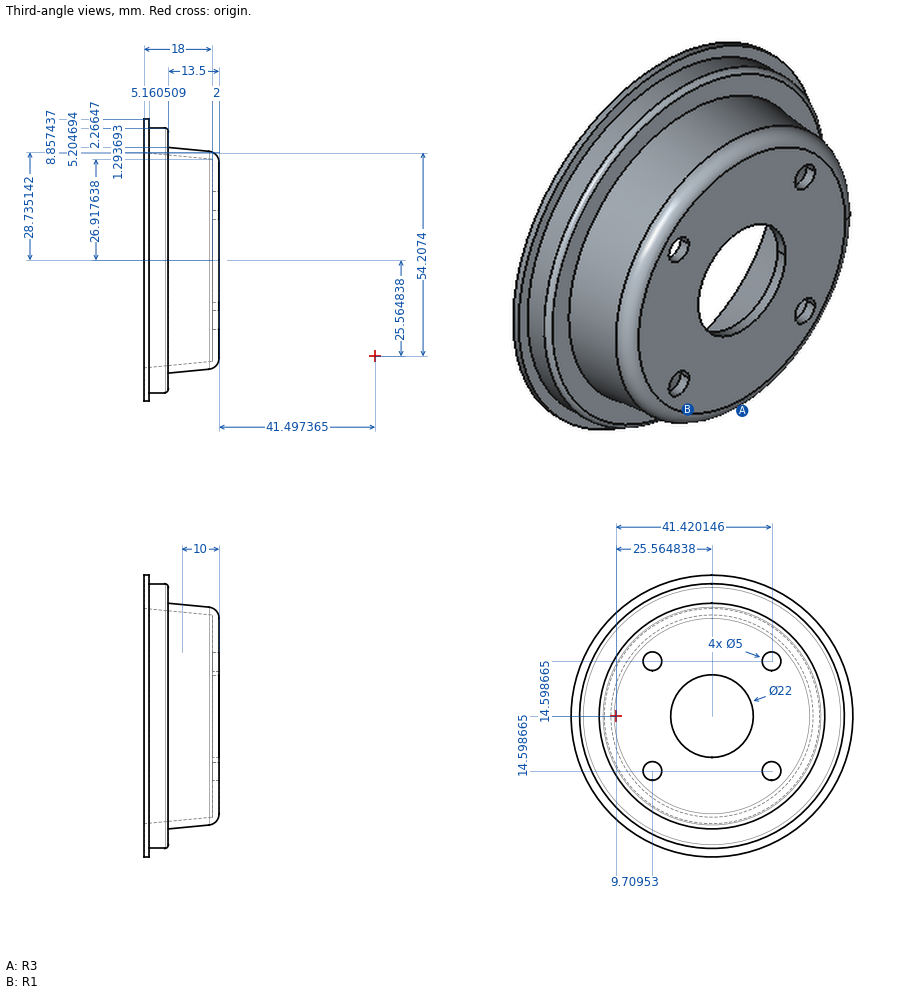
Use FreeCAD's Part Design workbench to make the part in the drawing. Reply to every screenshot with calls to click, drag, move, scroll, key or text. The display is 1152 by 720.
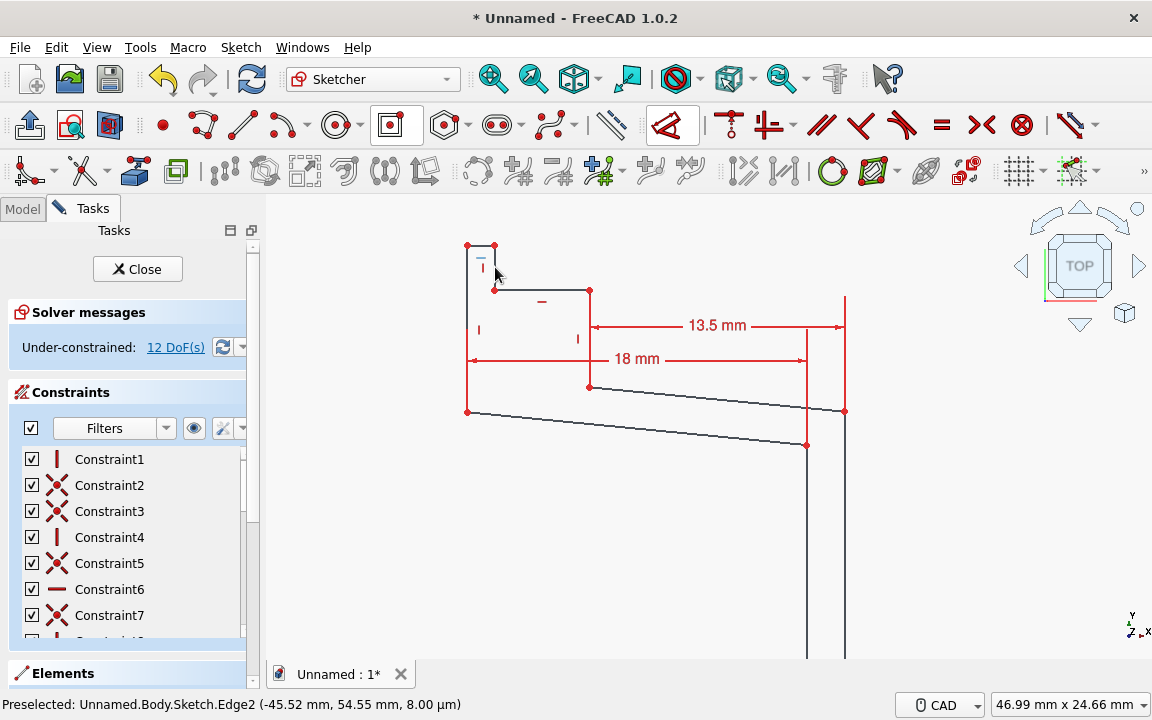
click(495, 268)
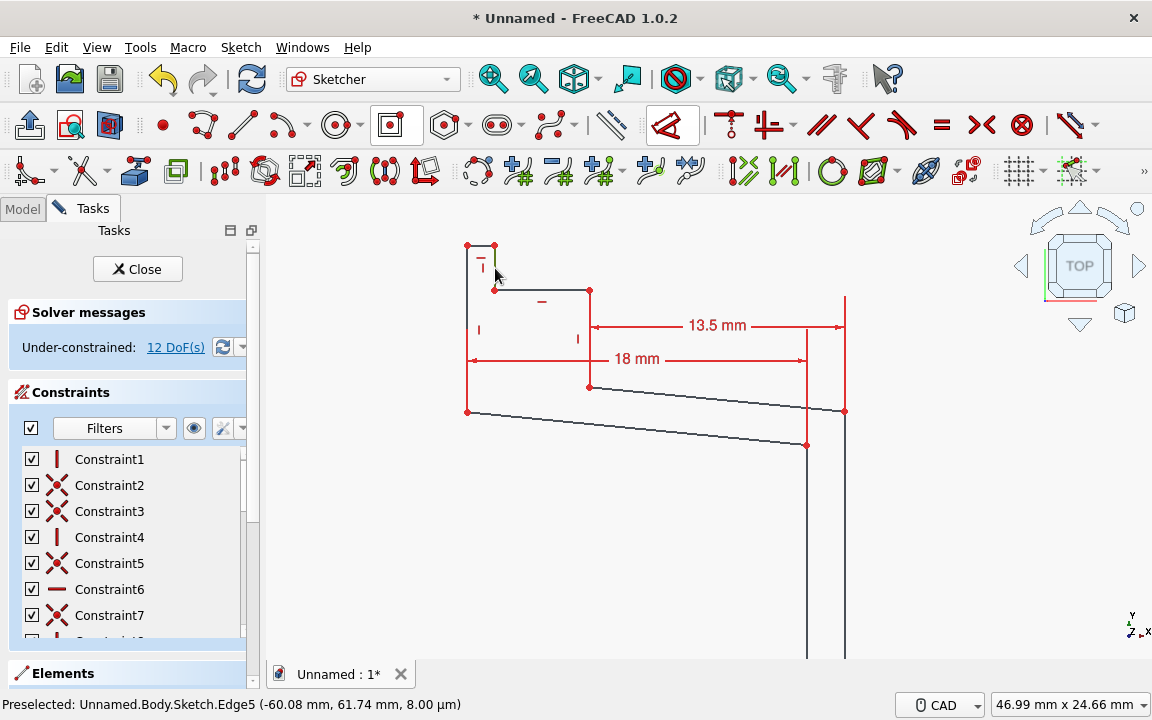
key(i)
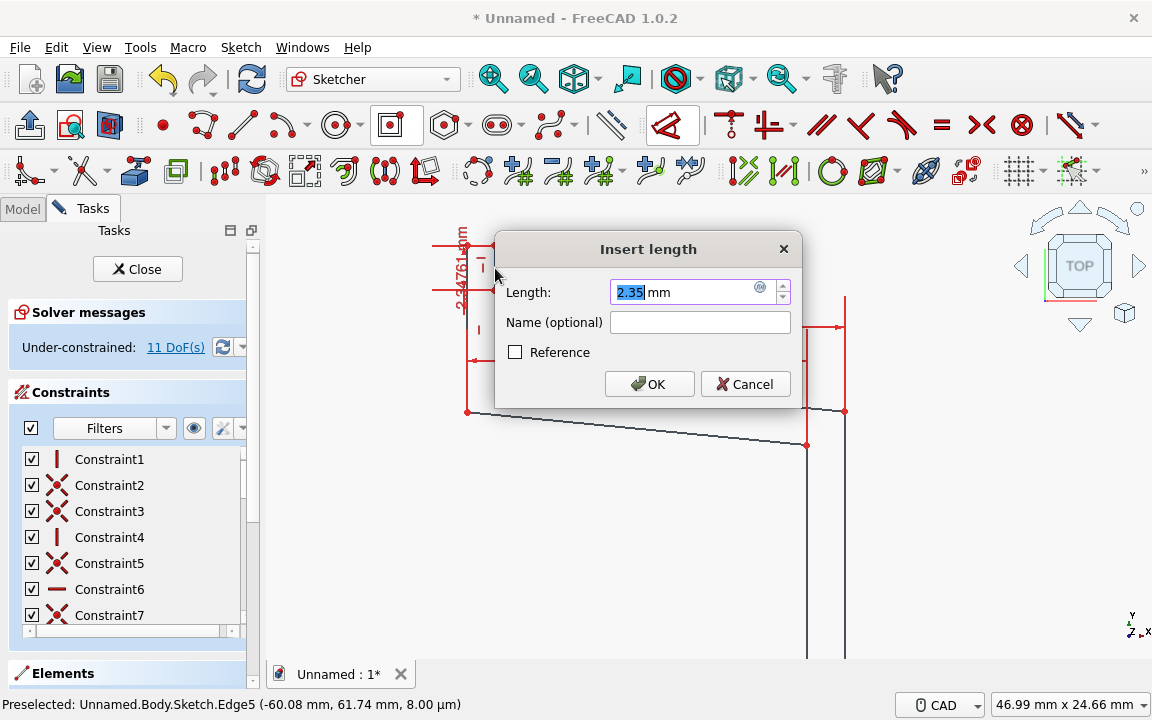
text(2.26647)
key(Return)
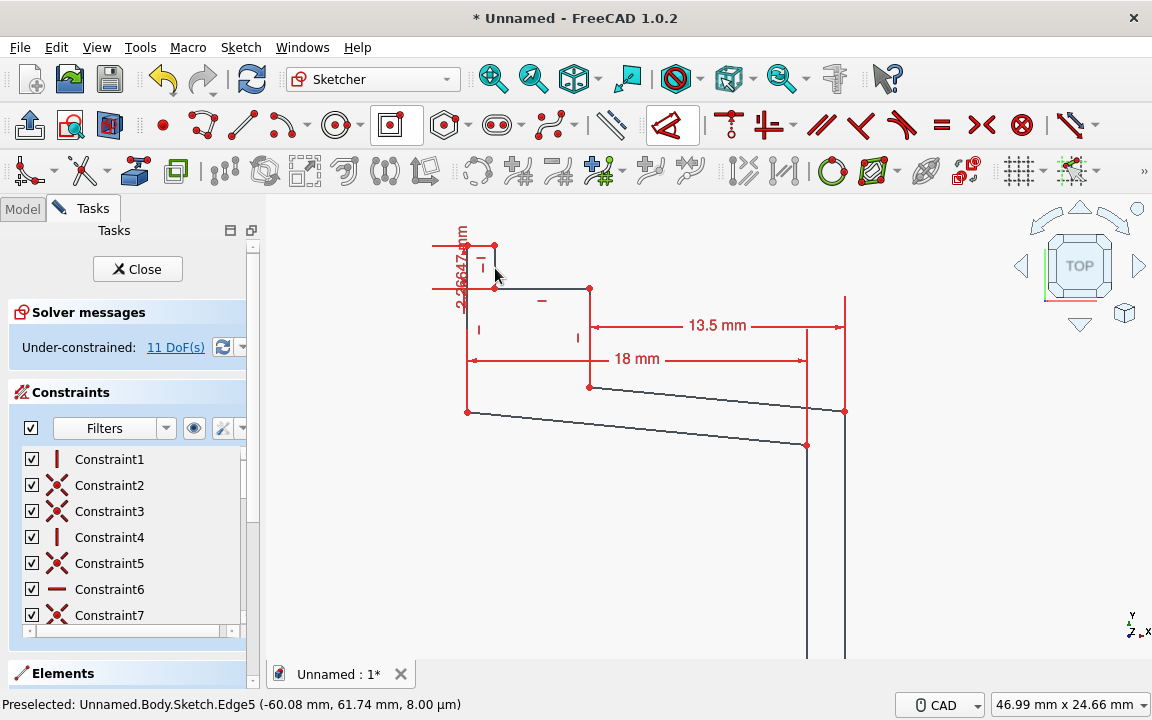
click(590, 358)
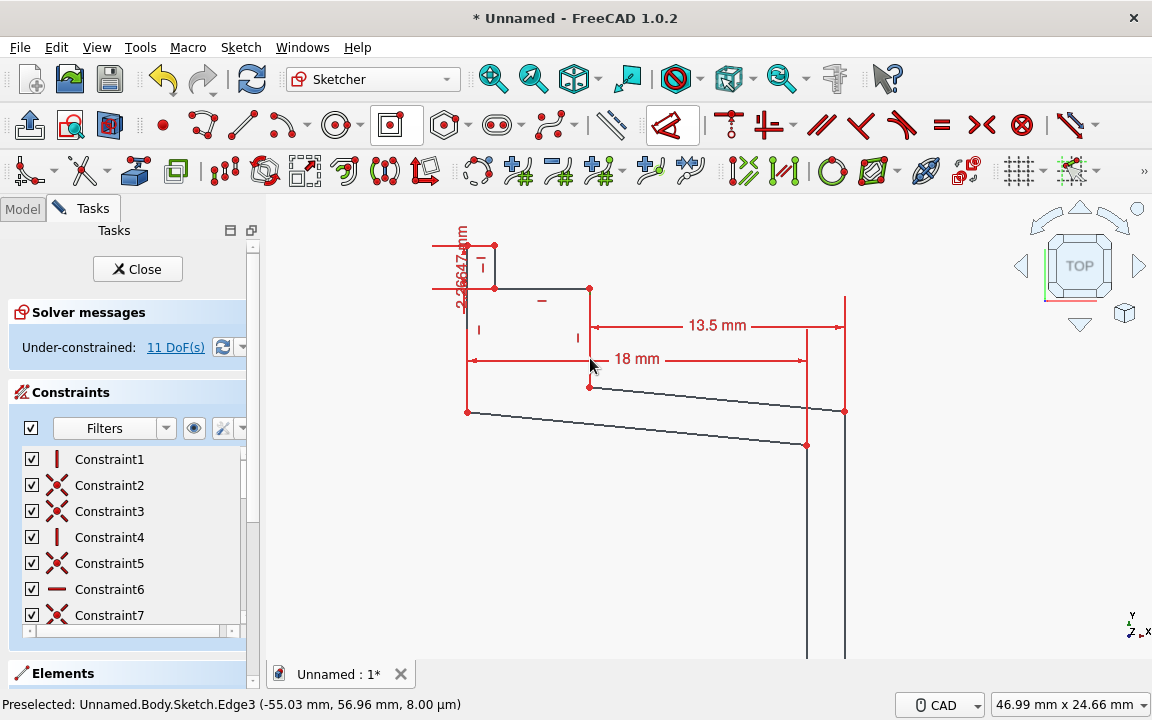
key(i)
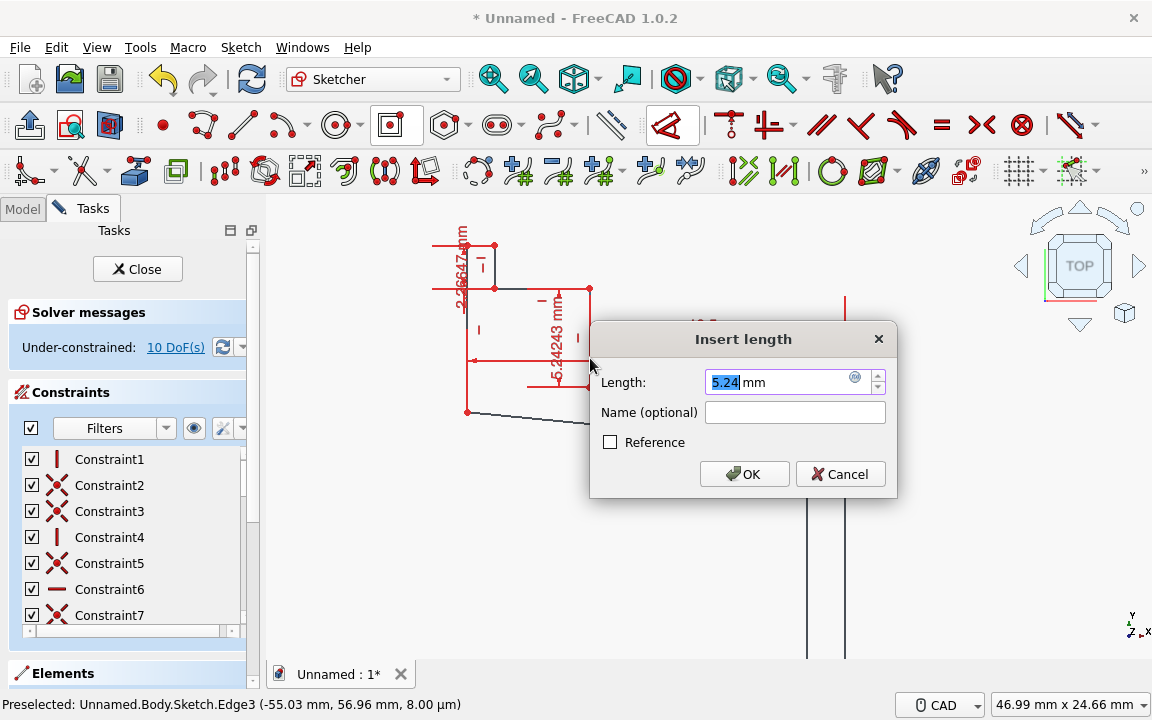
text(5.204694)
key(Return)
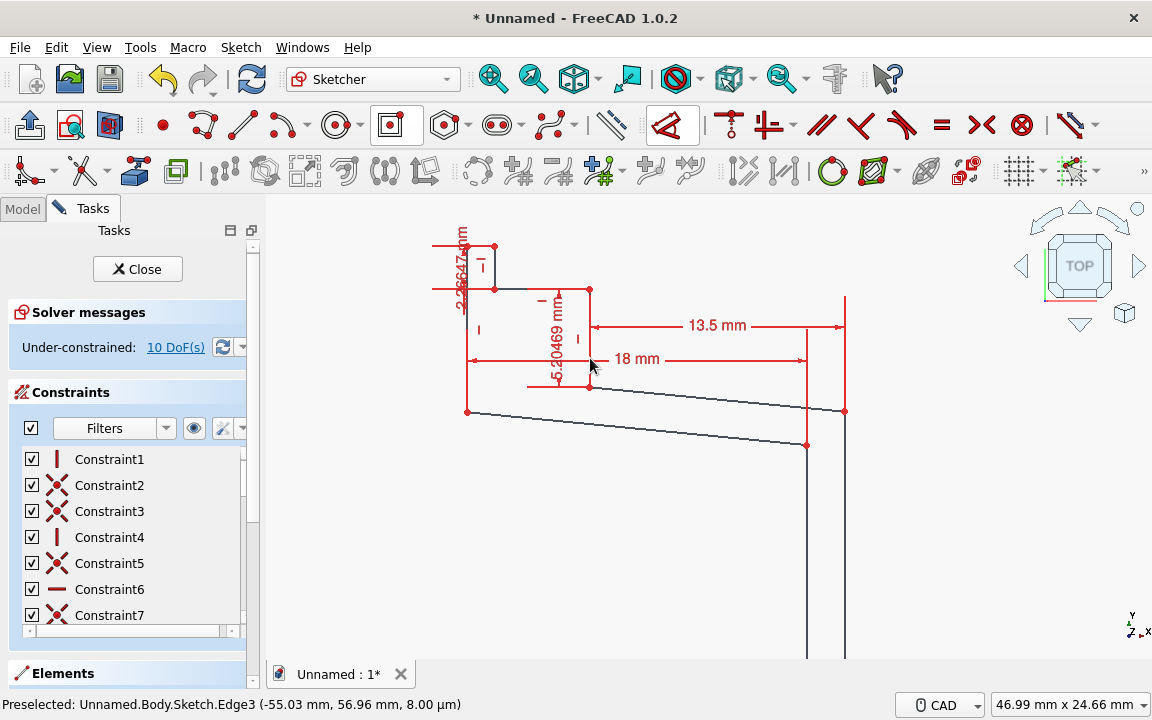
click(561, 289)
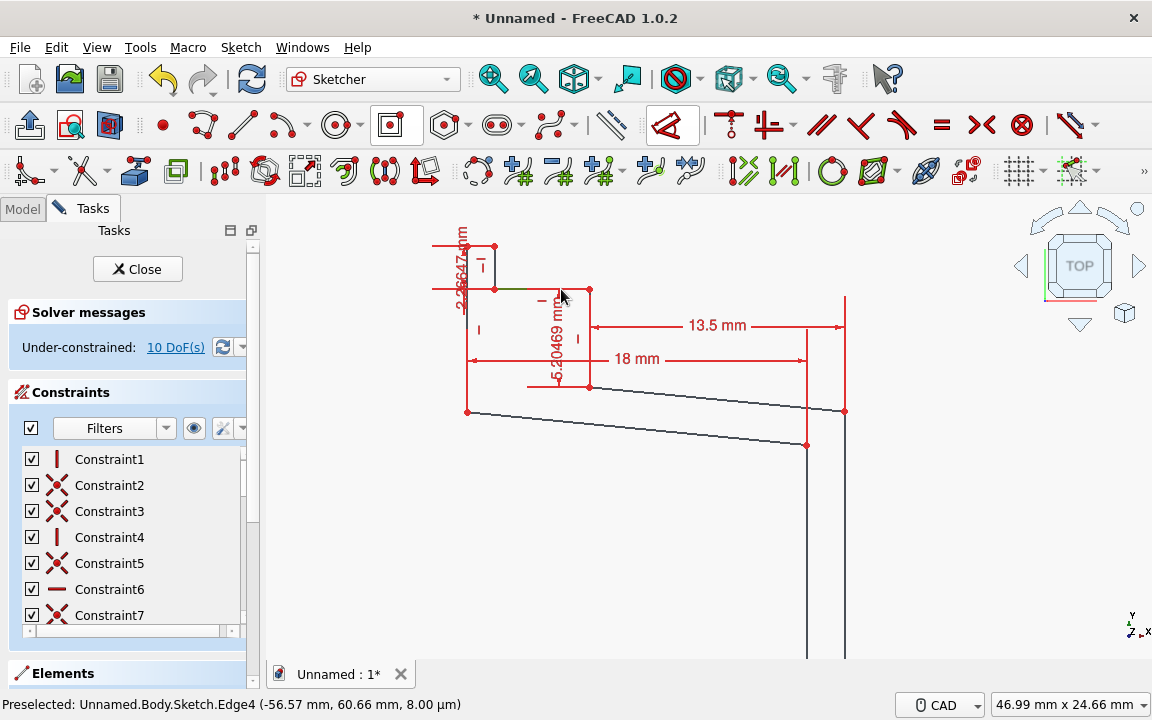
key(l)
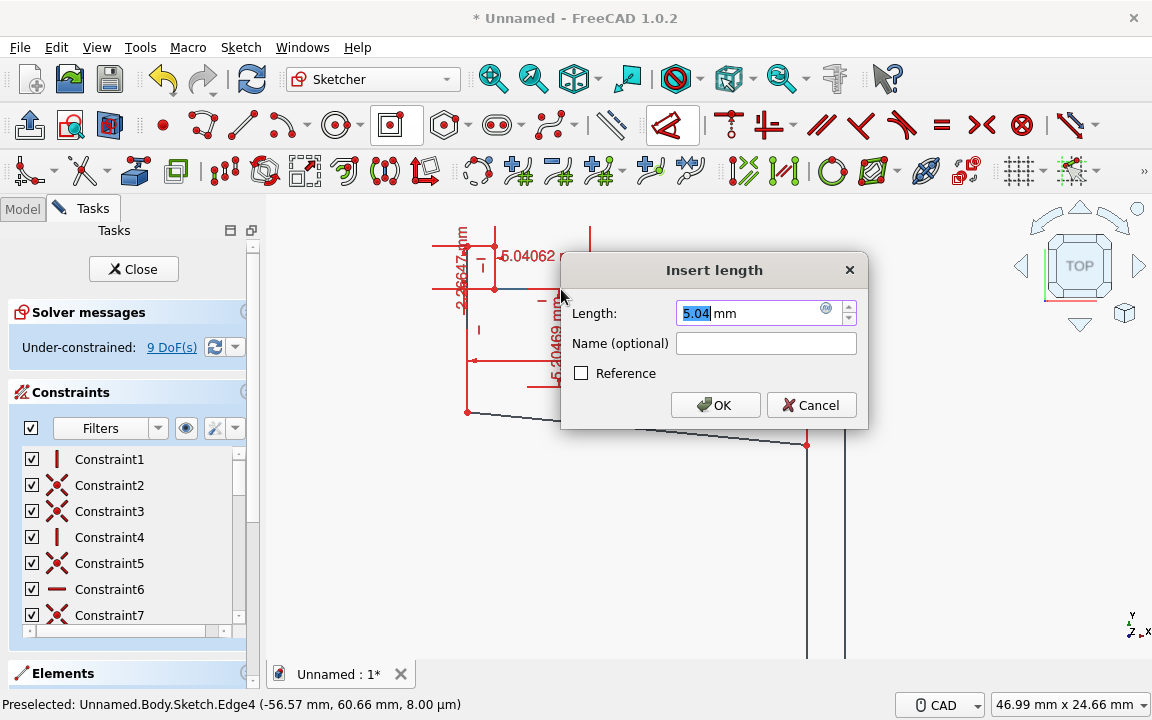
text(5.160509)
key(Return)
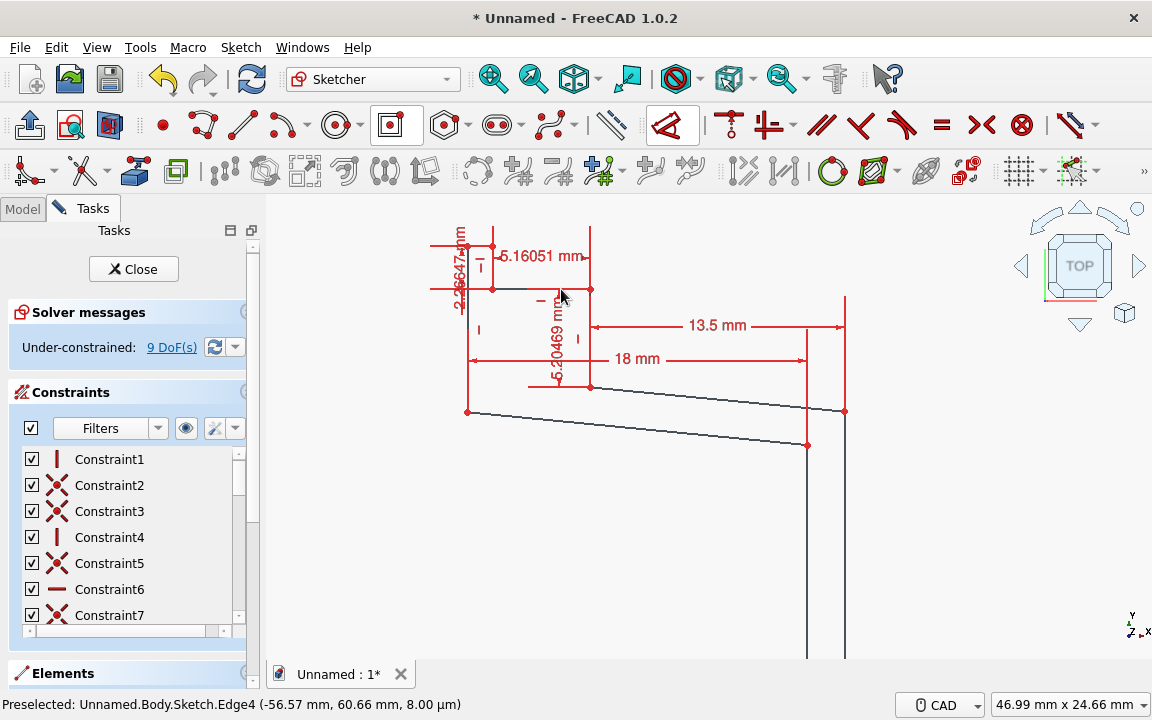
click(468, 363)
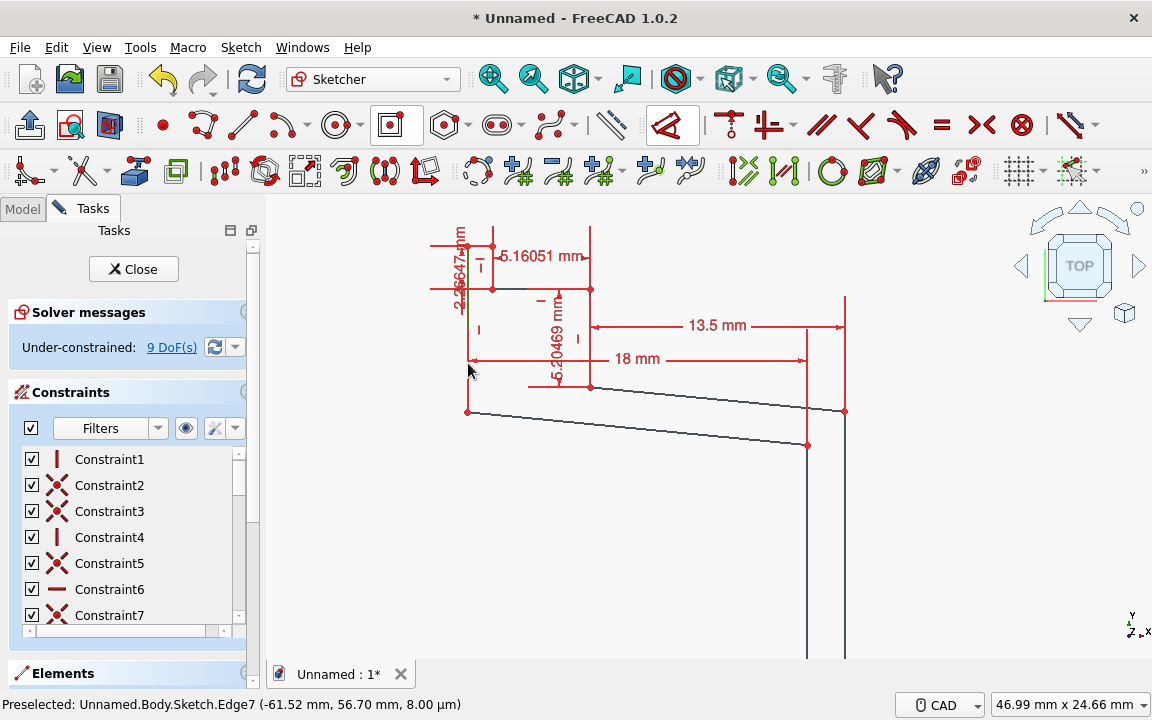
key(i)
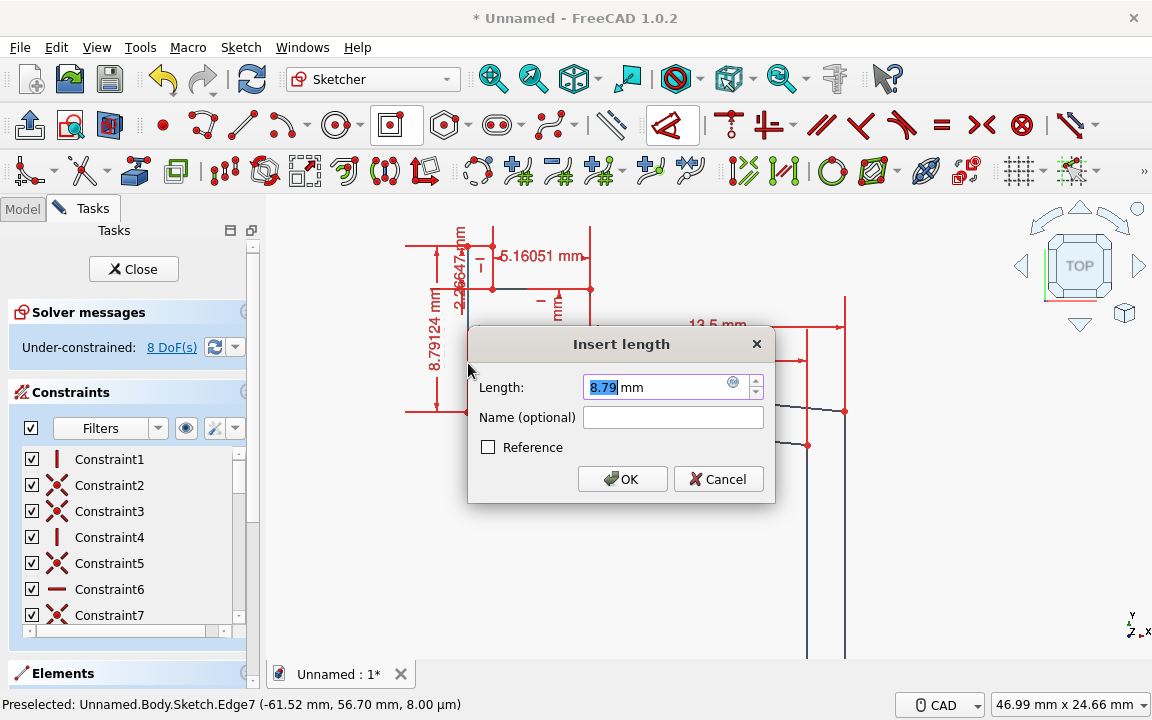
text(8.857437)
key(Return)